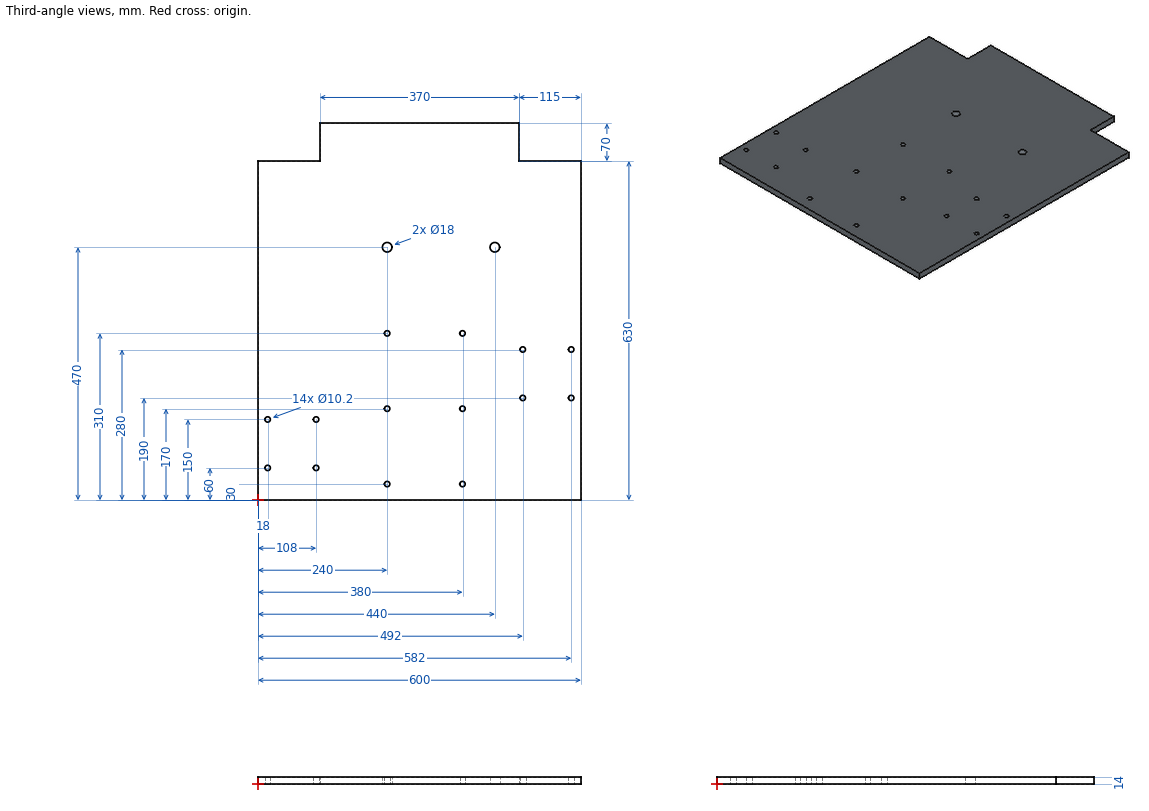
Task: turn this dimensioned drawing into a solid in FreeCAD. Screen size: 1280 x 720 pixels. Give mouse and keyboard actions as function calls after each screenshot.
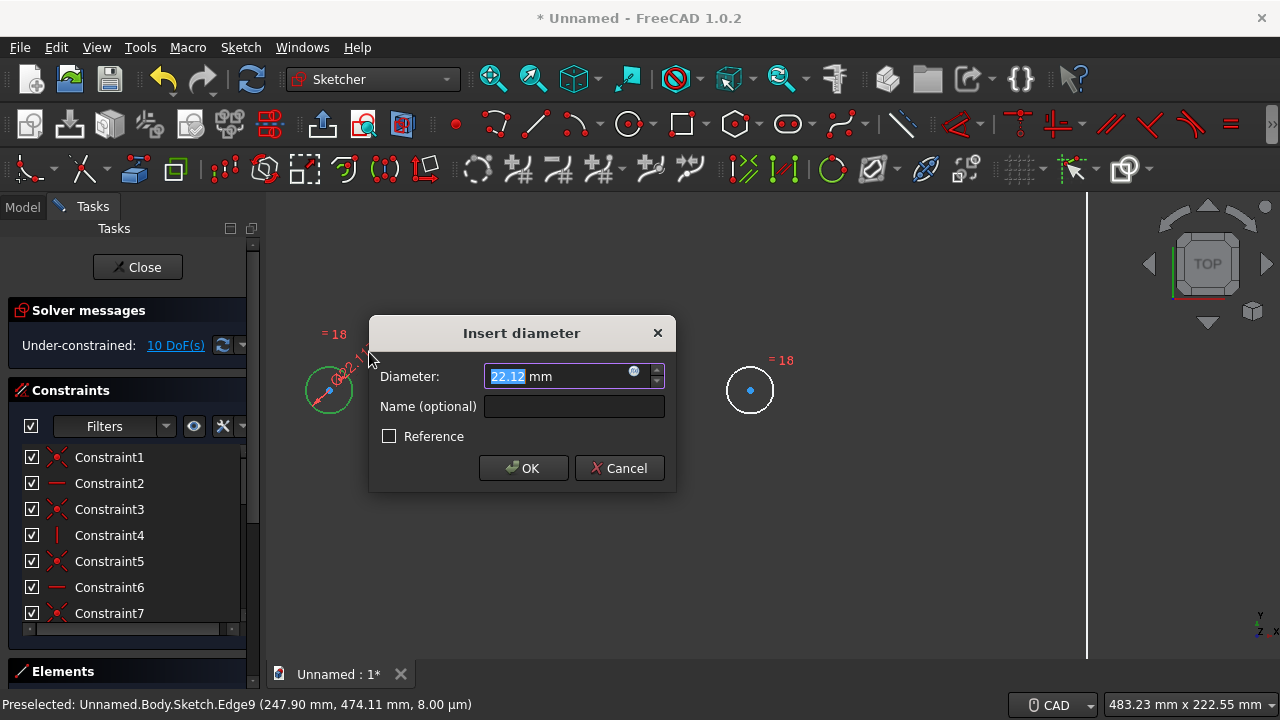
text(18)
key(Return)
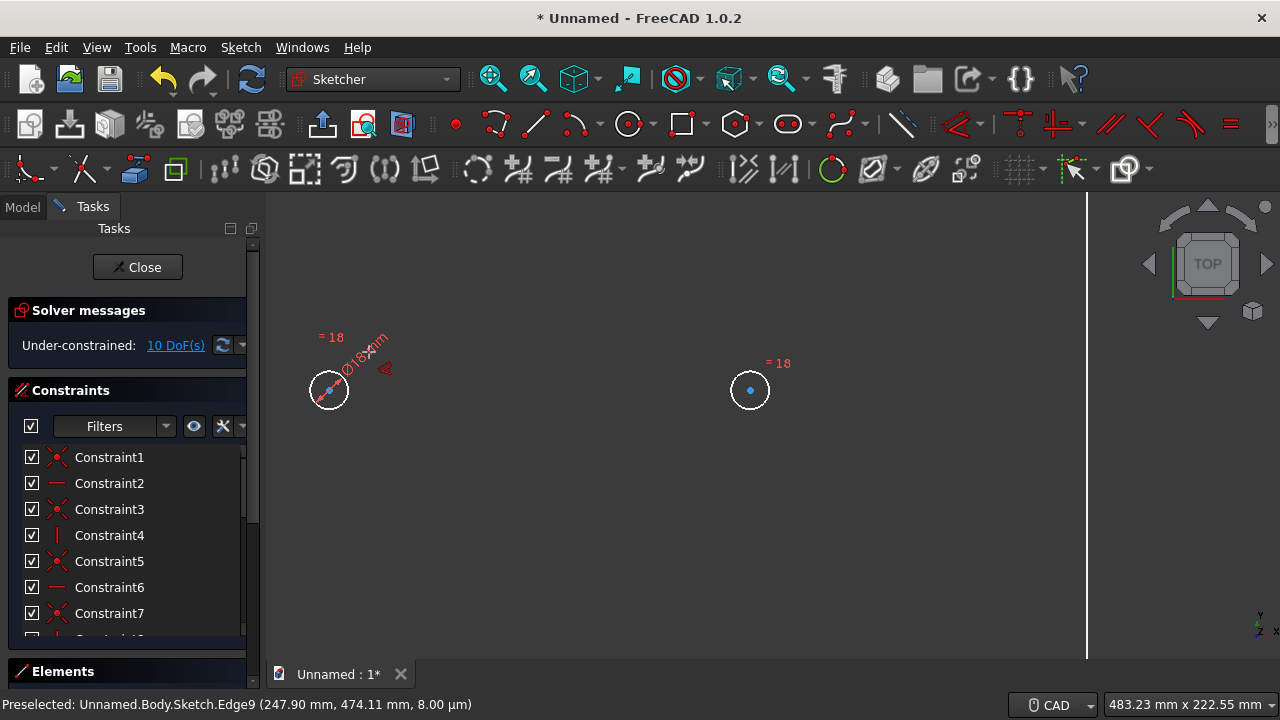
scroll(767, 372, down, 8)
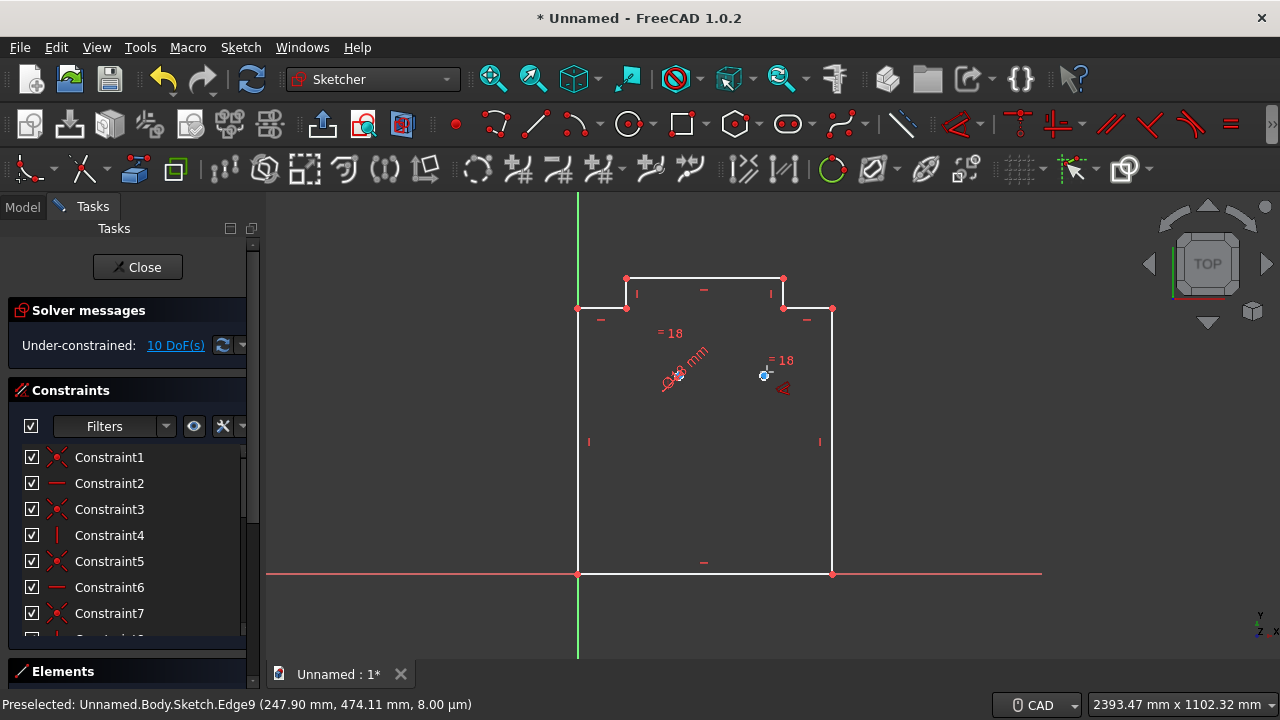
scroll(783, 299, up, 3)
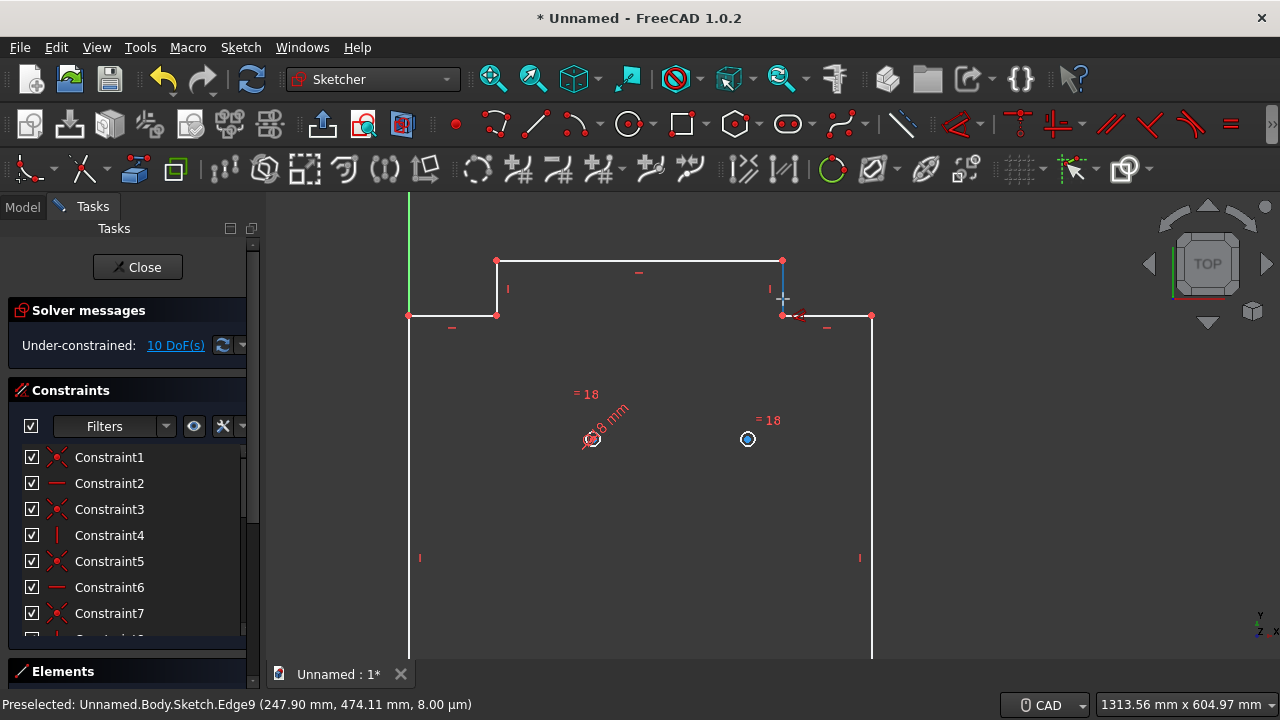
click(783, 299)
click(817, 288)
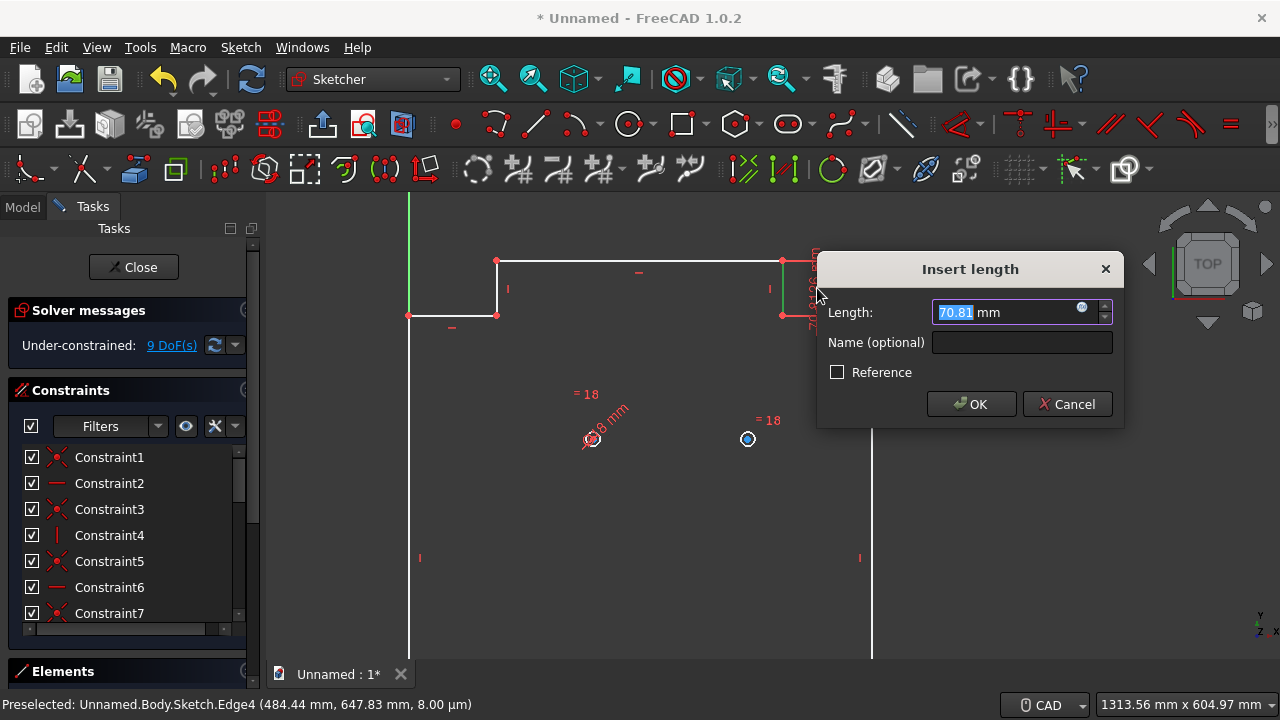
text(70)
key(Return)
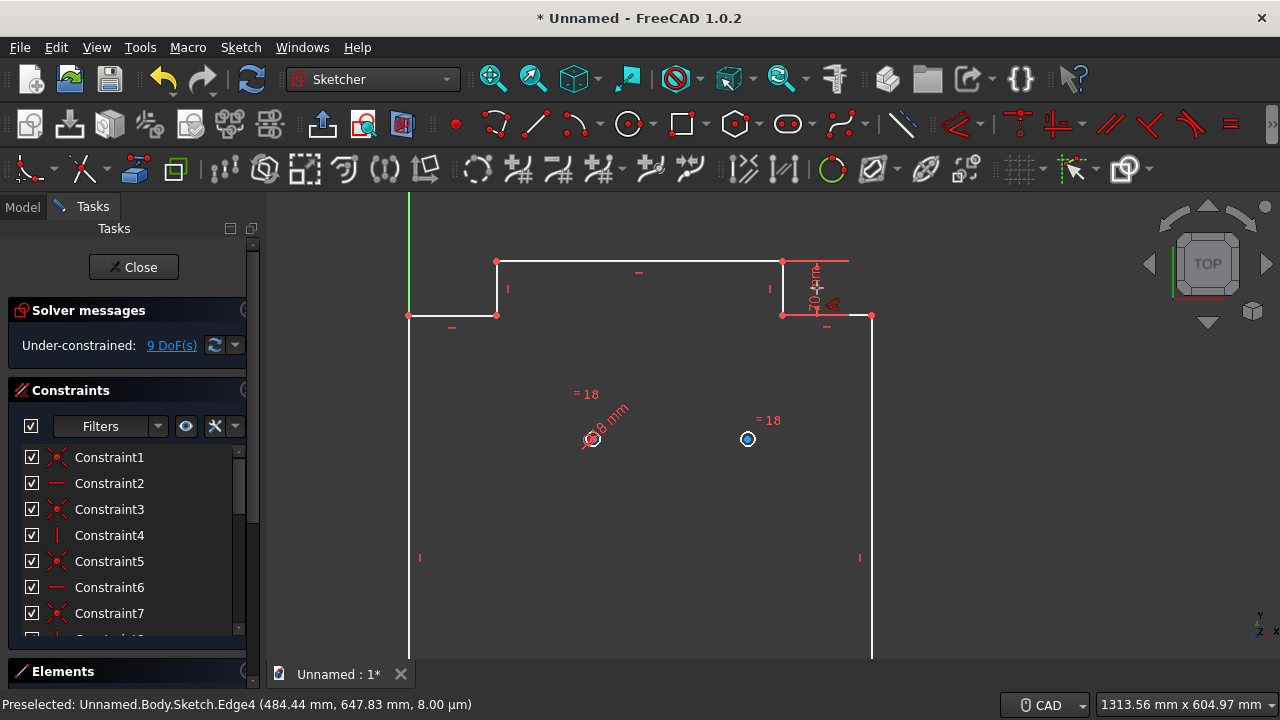
click(497, 278)
click(463, 288)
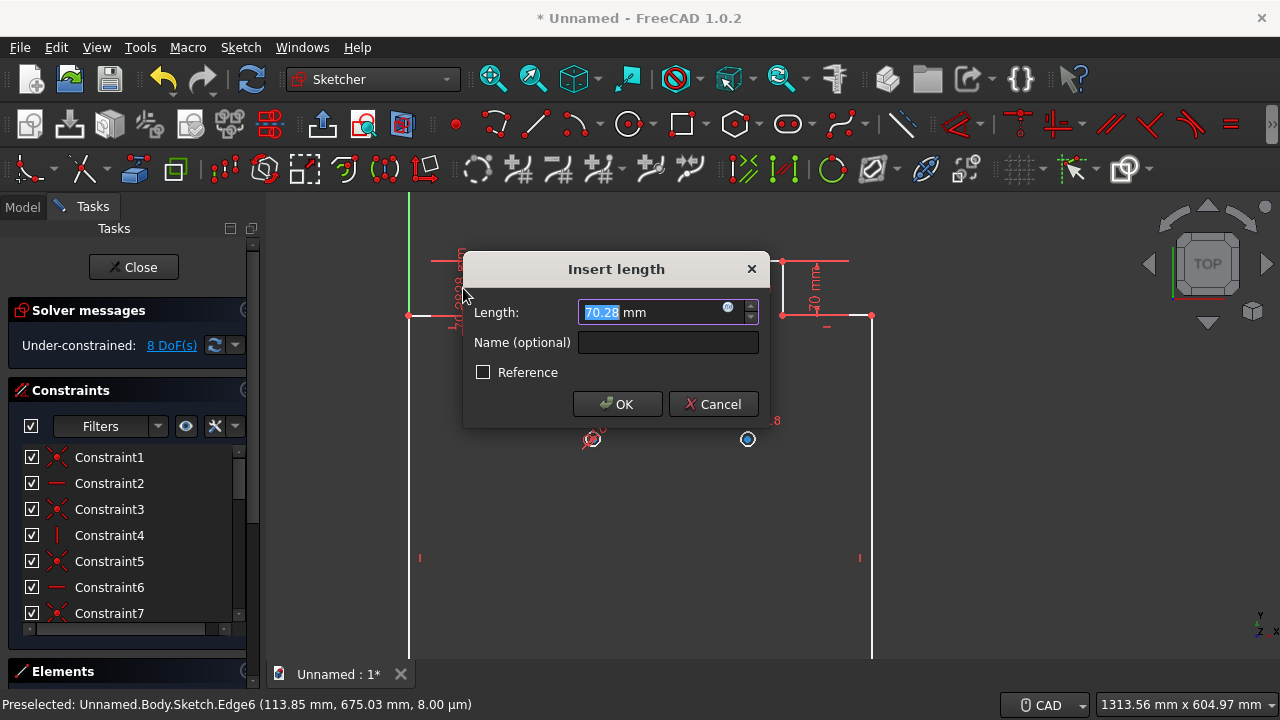
text(70)
key(Return)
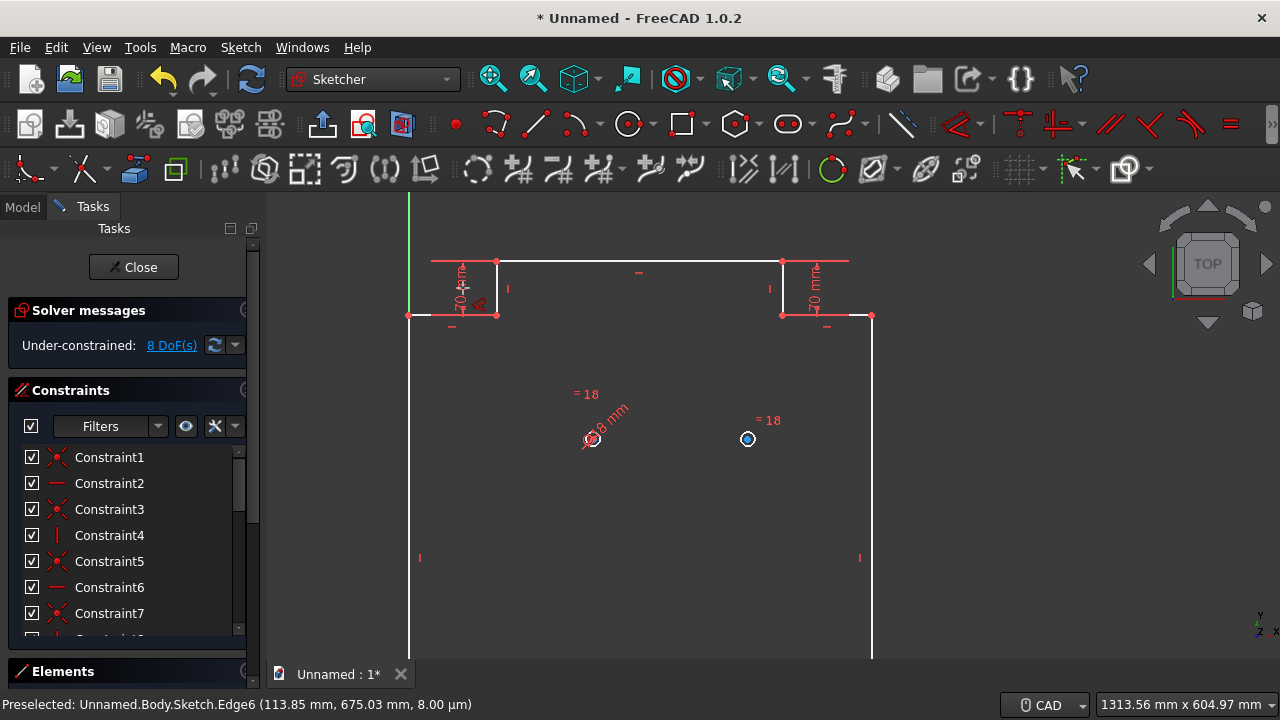
scroll(783, 299, down, 3)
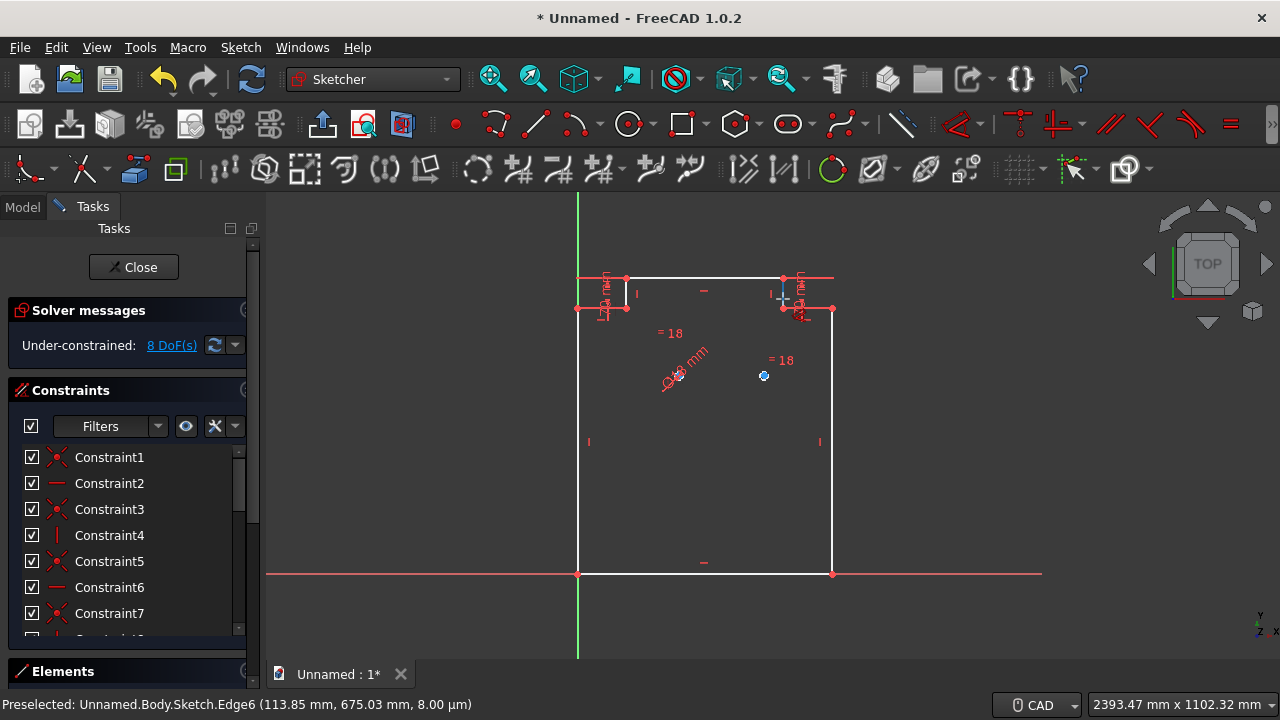
click(654, 574)
click(705, 608)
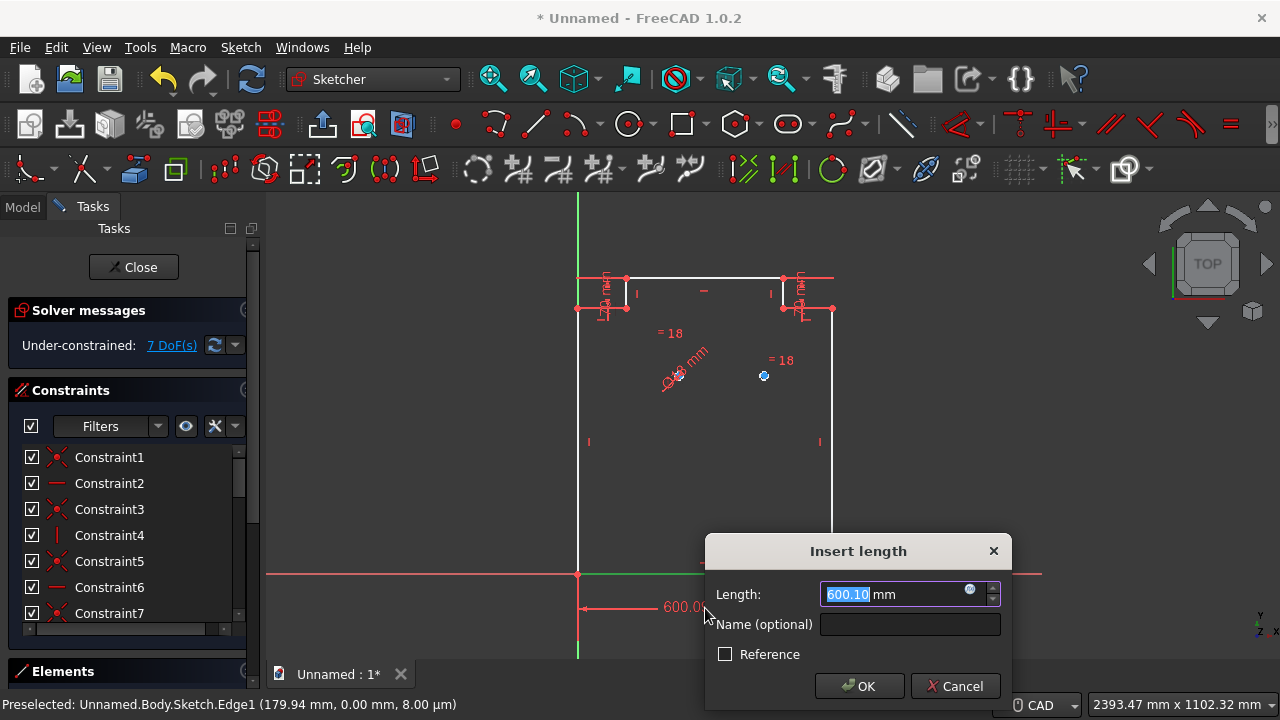
text(600)
key(Return)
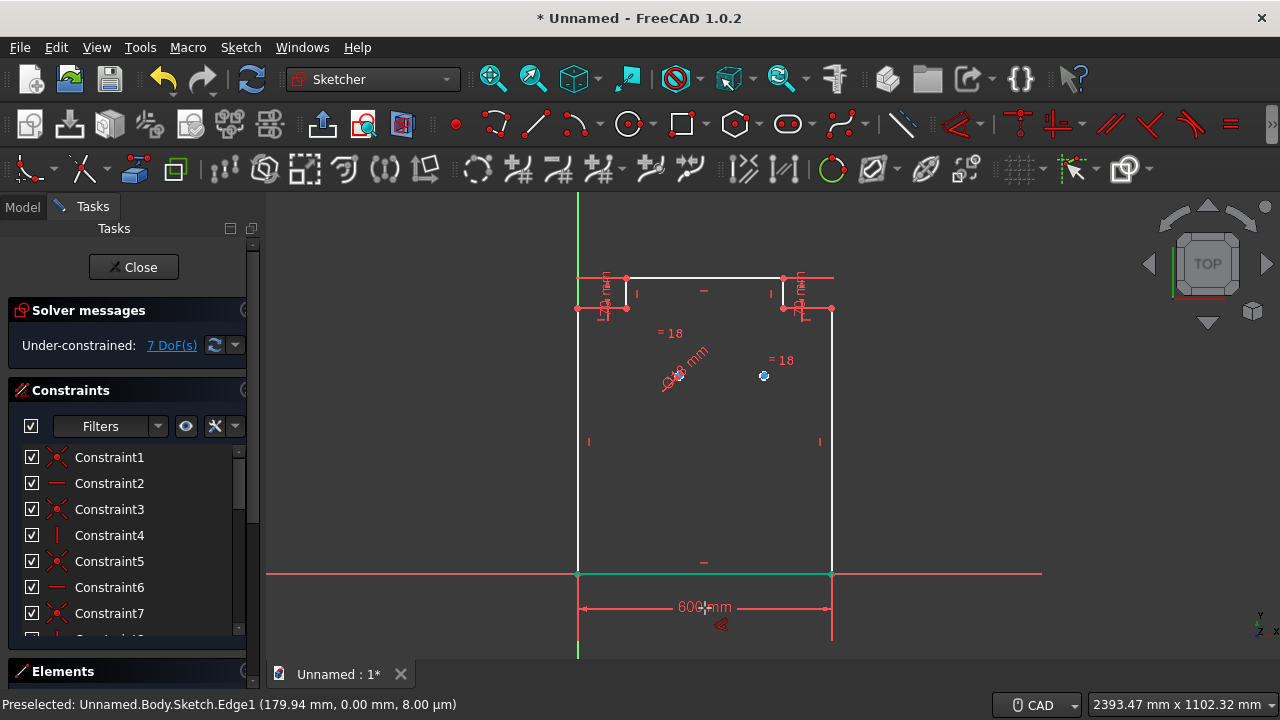
click(832, 494)
click(866, 441)